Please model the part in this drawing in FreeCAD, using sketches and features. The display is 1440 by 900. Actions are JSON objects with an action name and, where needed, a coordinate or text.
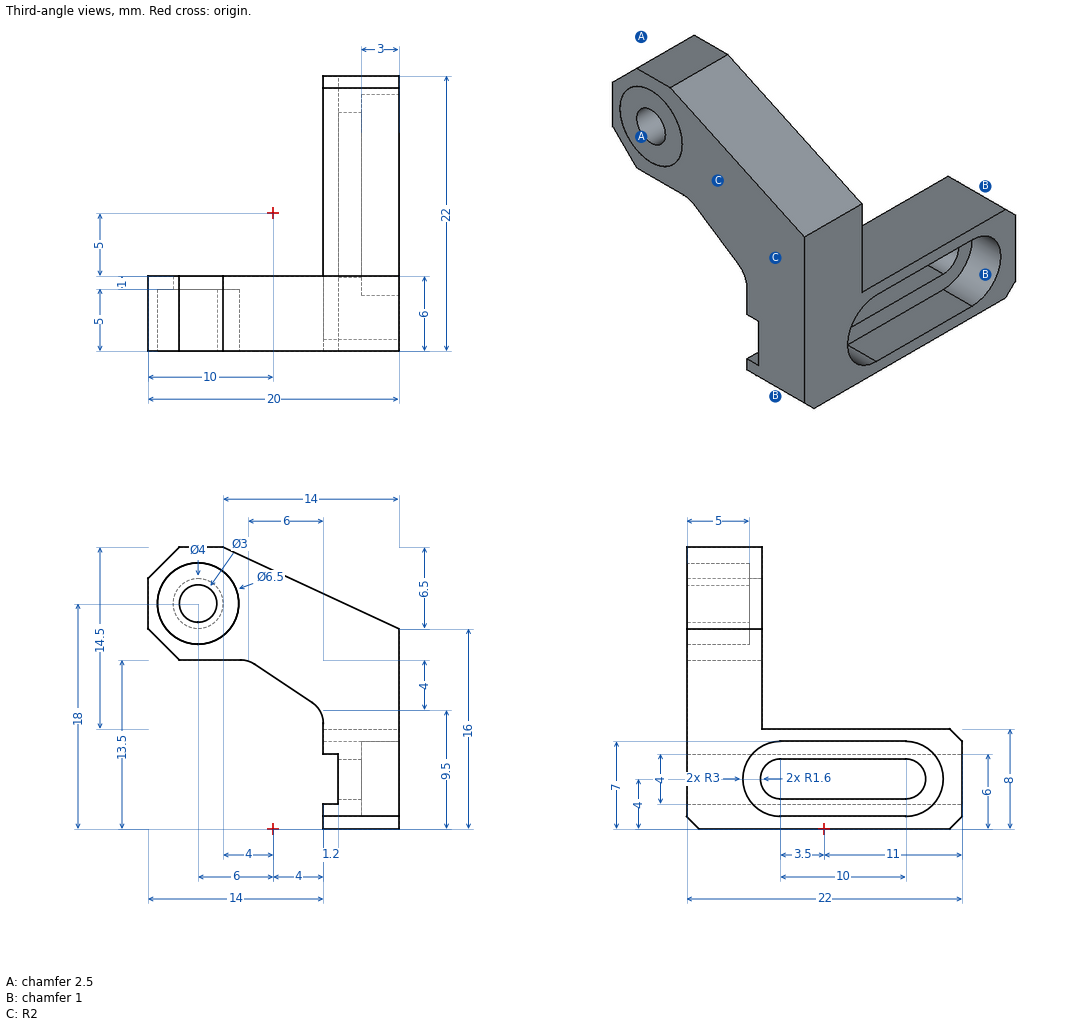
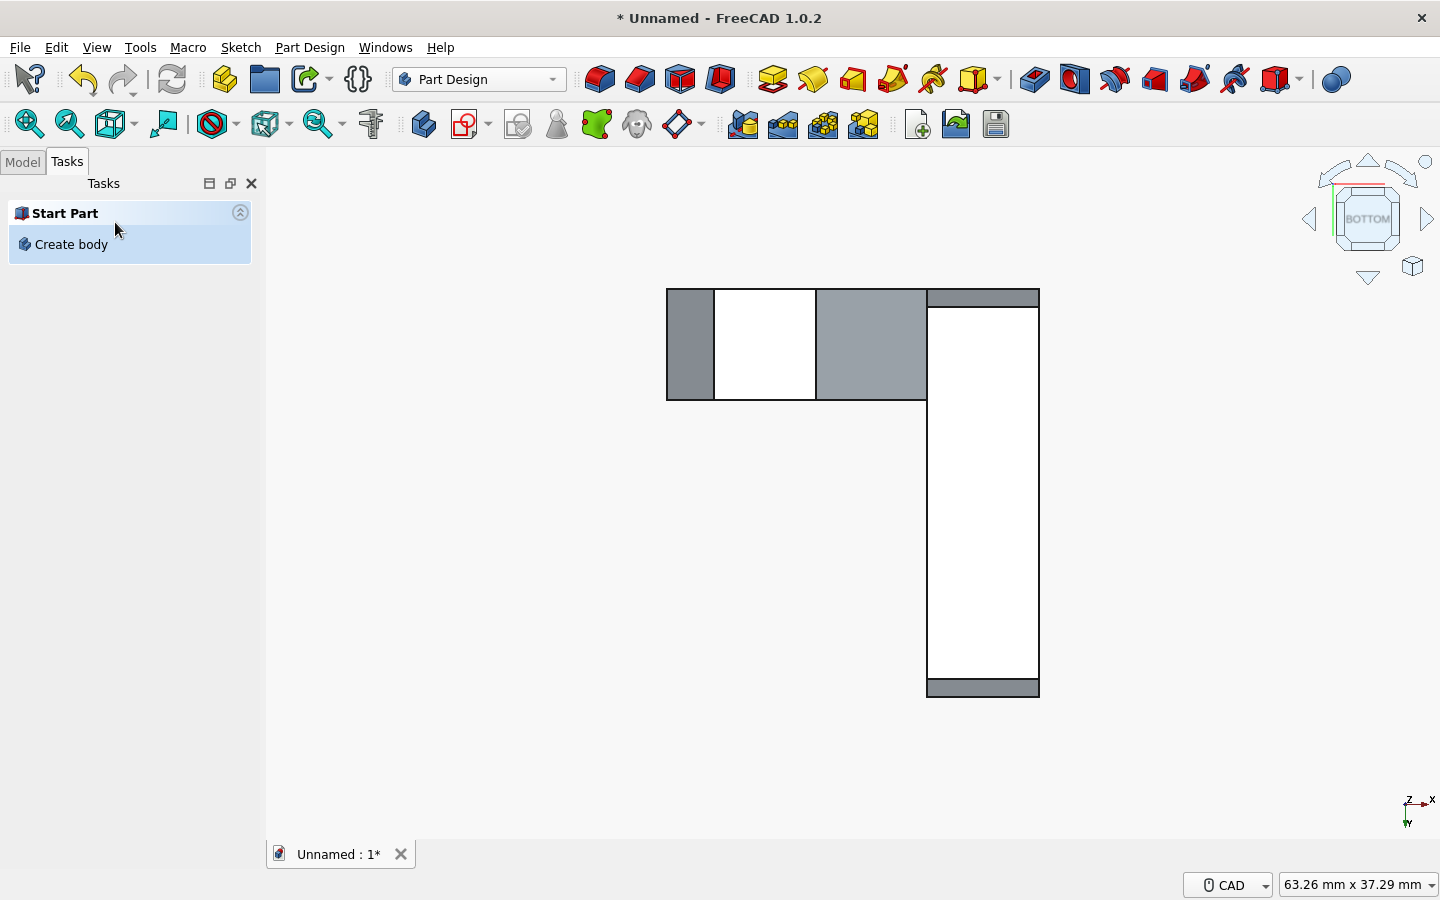
{"action": "key", "text": "4"}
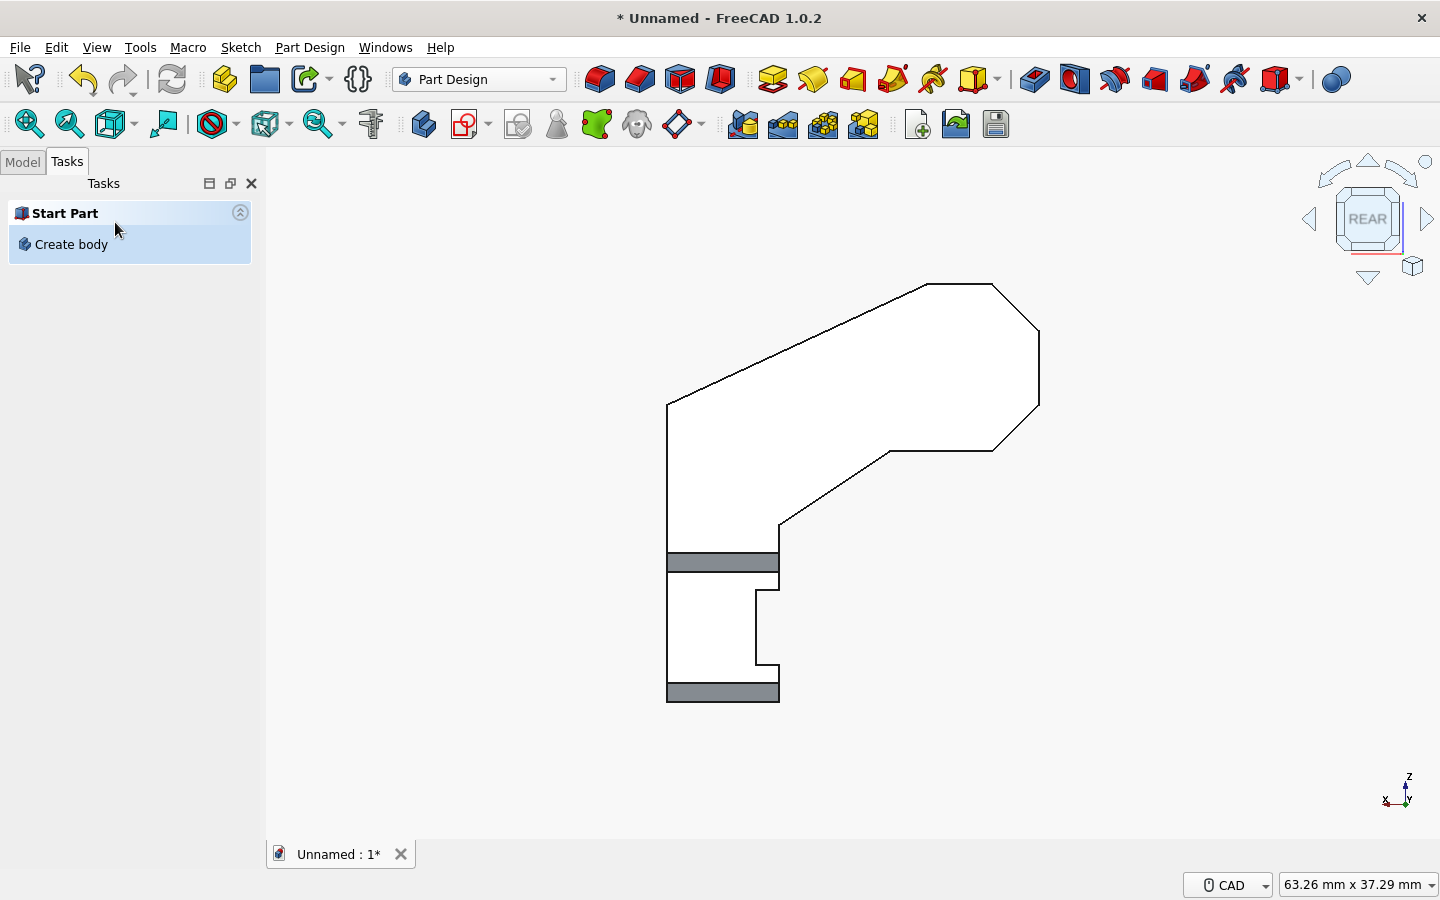
{"action": "key", "text": "6"}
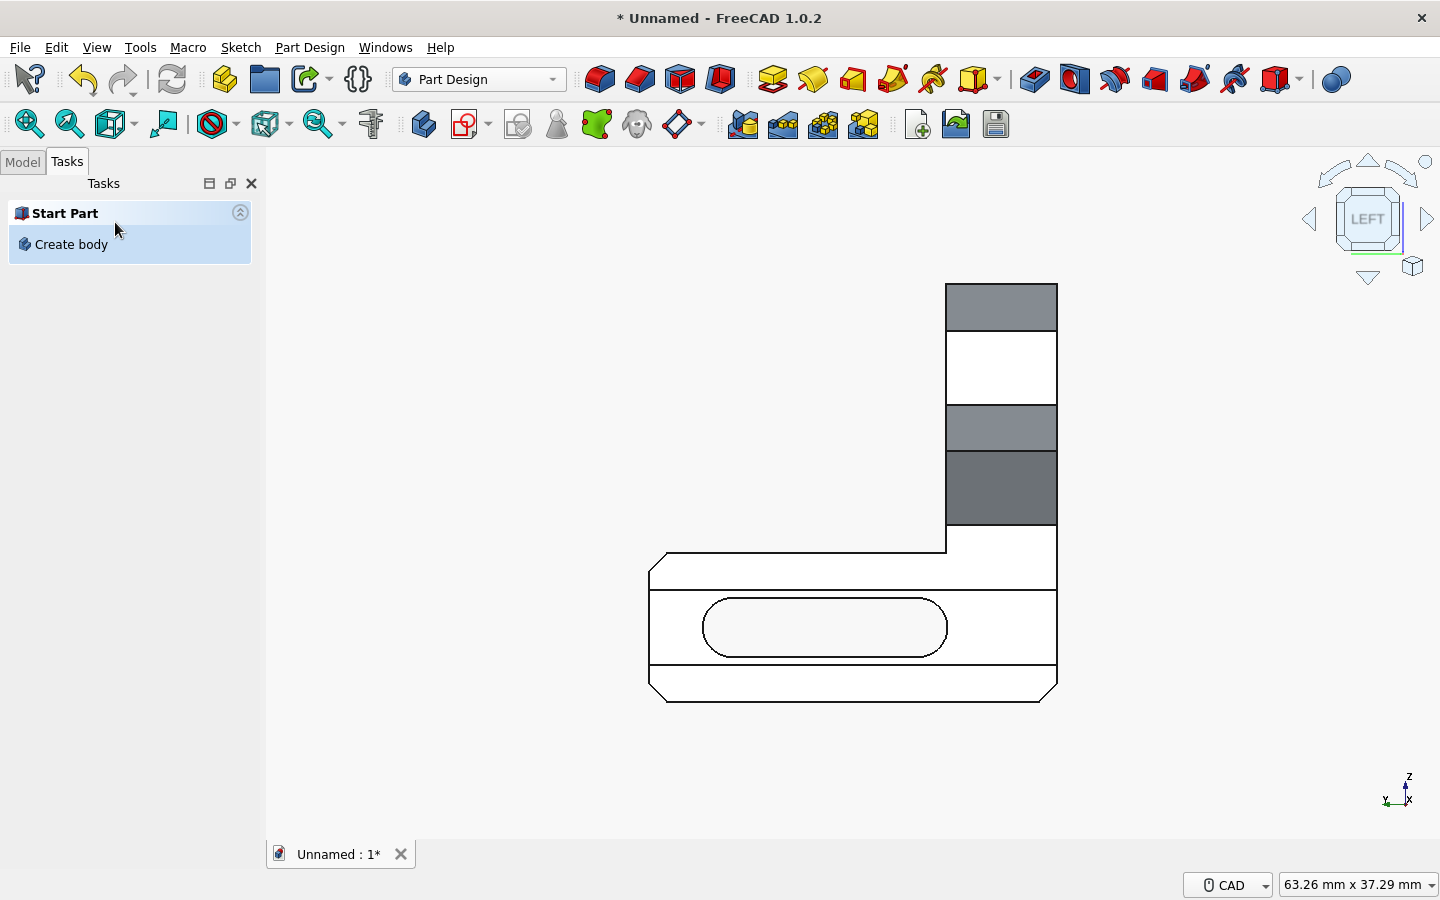
{"action": "key", "text": "v 3"}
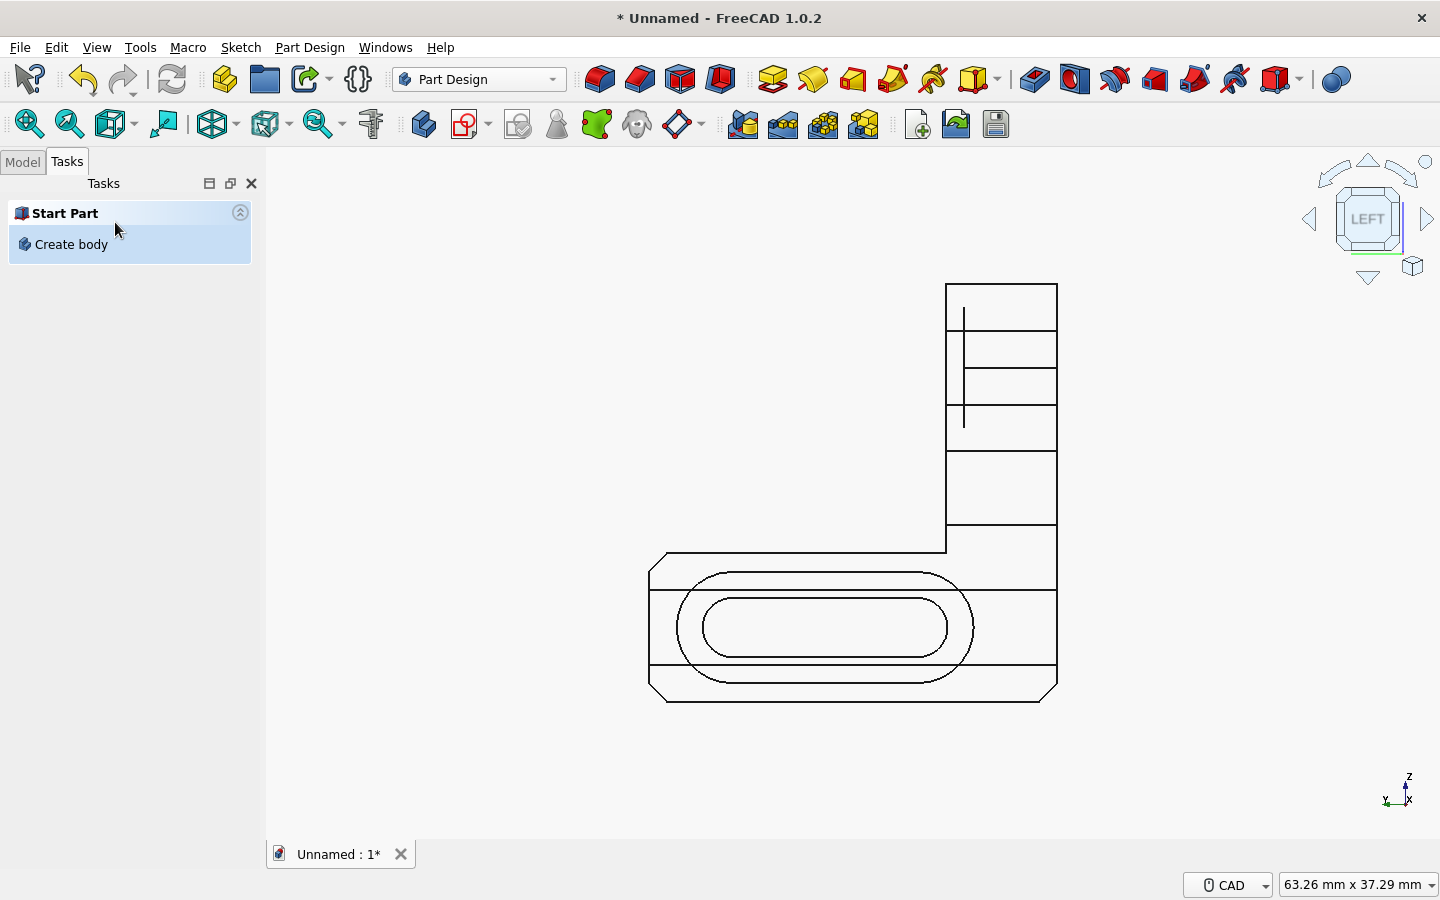
{"action": "key", "text": "0"}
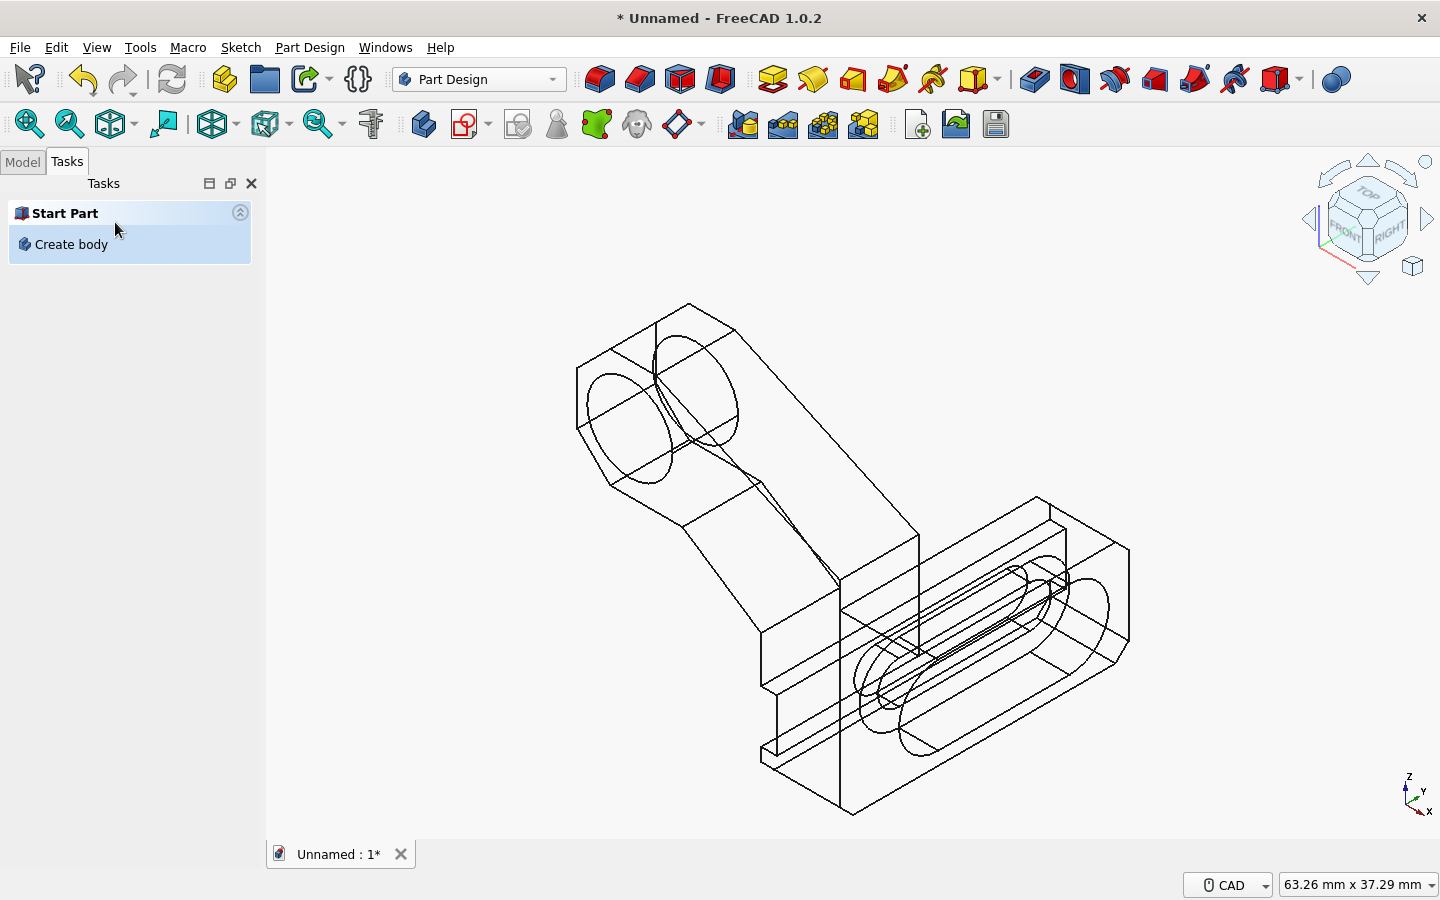
{"action": "left_click", "coordinate": [722, 503]}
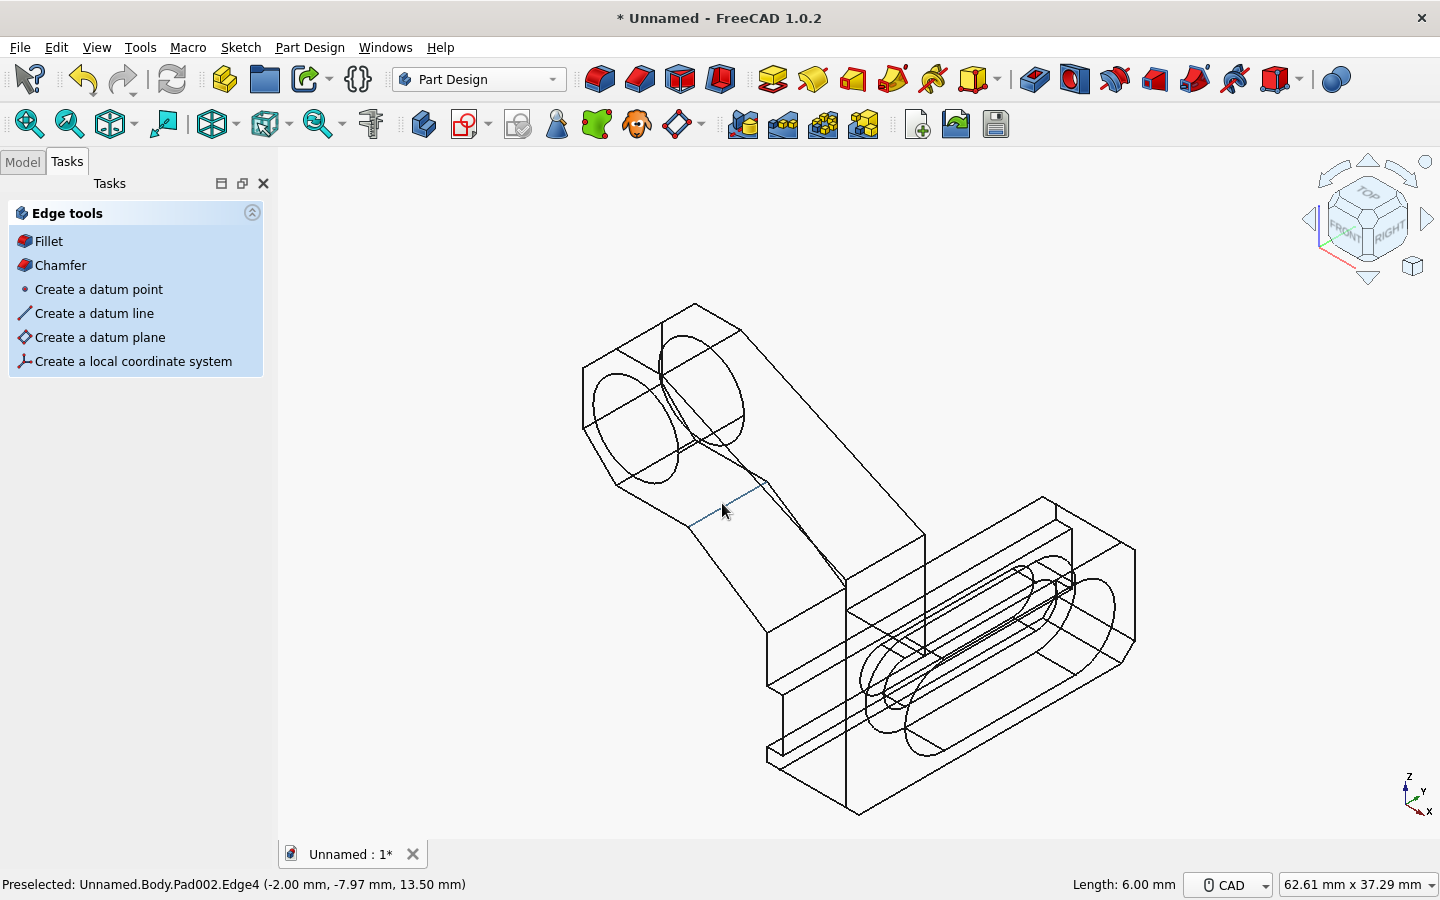
{"action": "left_click", "coordinate": [807, 609], "text": "ctrl"}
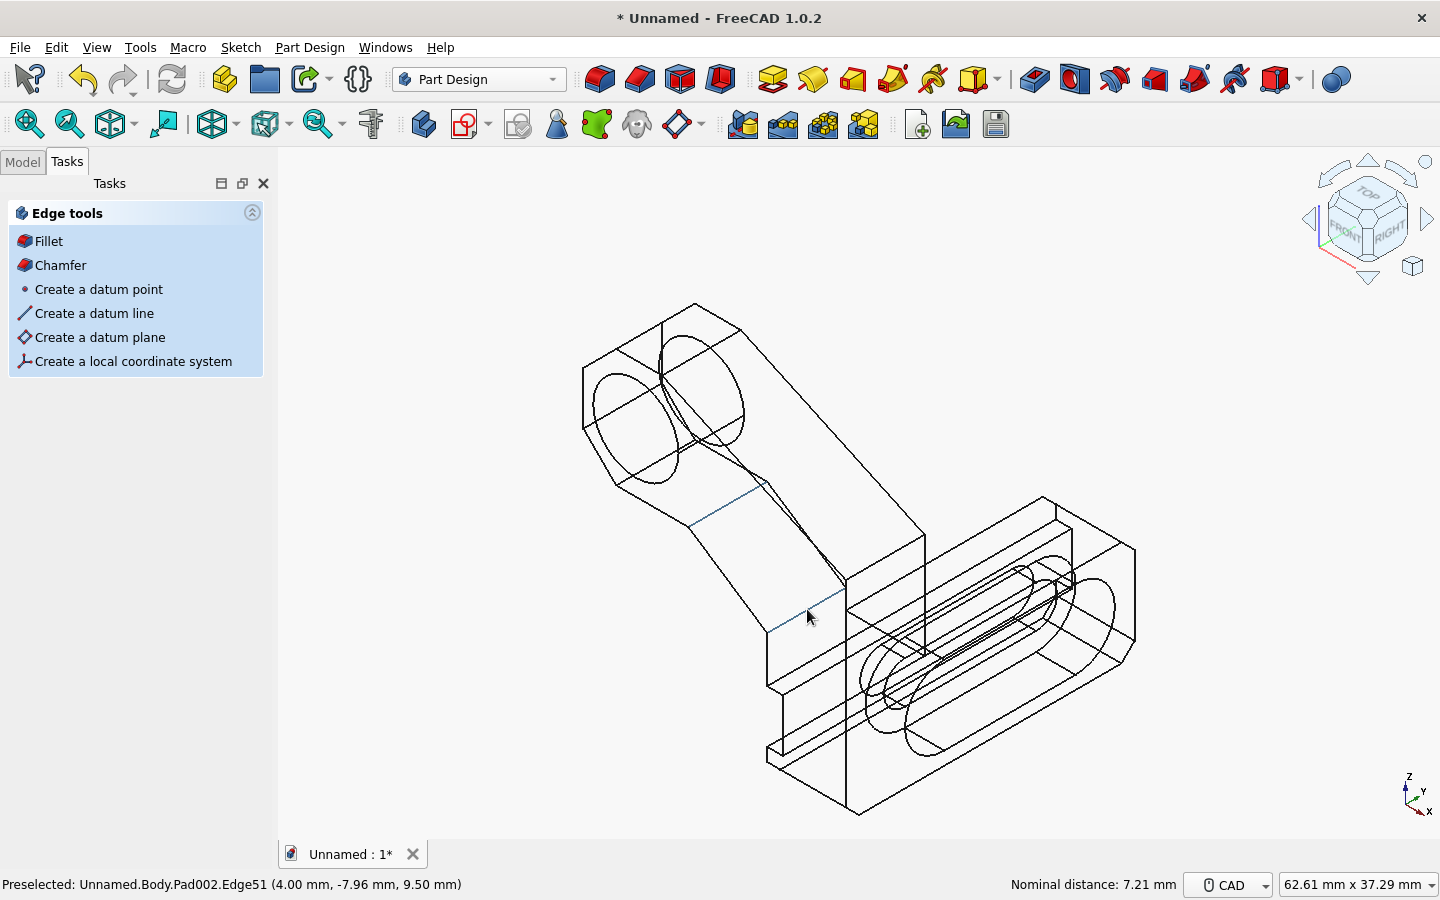
{"action": "key", "text": "v 1"}